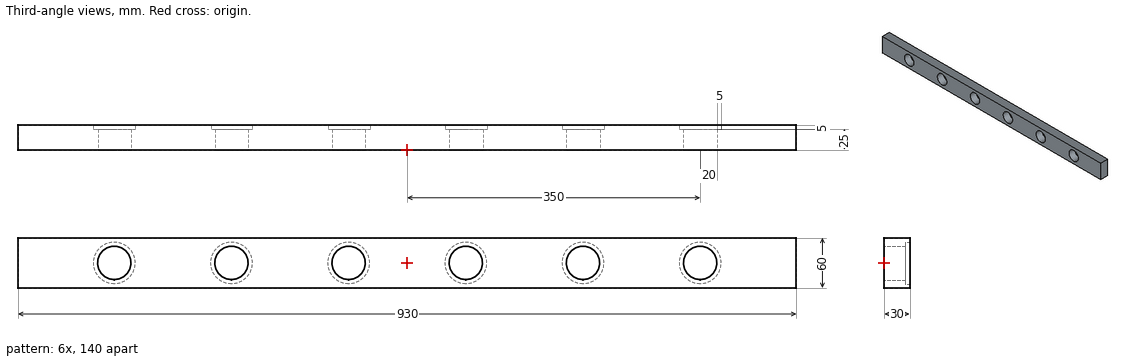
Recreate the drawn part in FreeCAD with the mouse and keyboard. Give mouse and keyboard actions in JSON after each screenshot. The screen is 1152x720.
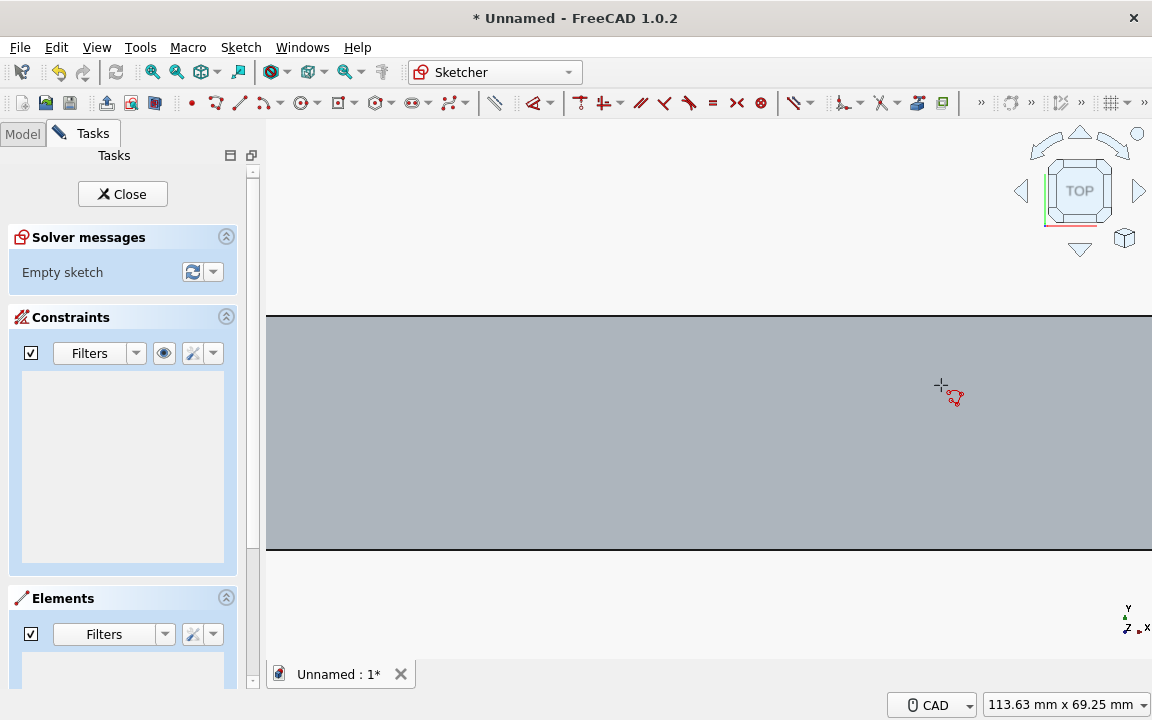
{"action": "left_click", "coordinate": [537, 550]}
{"action": "left_click", "coordinate": [693, 541]}
{"action": "left_click", "coordinate": [693, 355]}
{"action": "left_click", "coordinate": [732, 355]}
{"action": "left_click", "coordinate": [732, 316]}
{"action": "left_click", "coordinate": [537, 316]}
{"action": "left_click", "coordinate": [537, 551]}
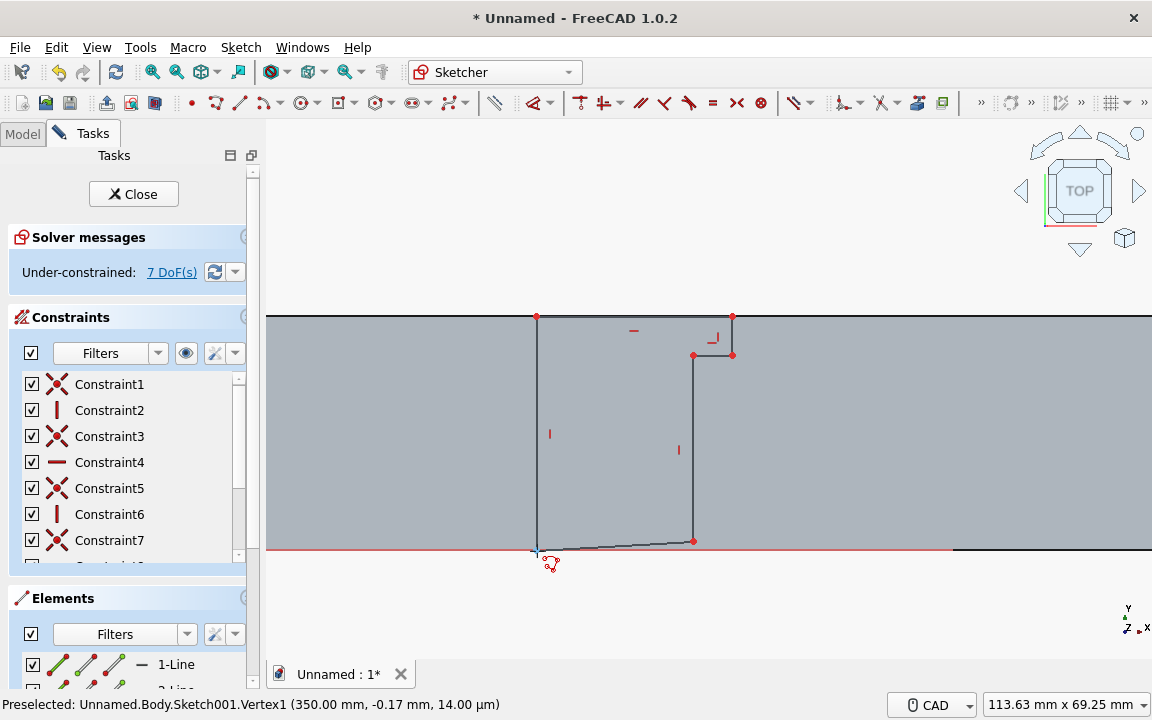
{"action": "key", "text": "g l"}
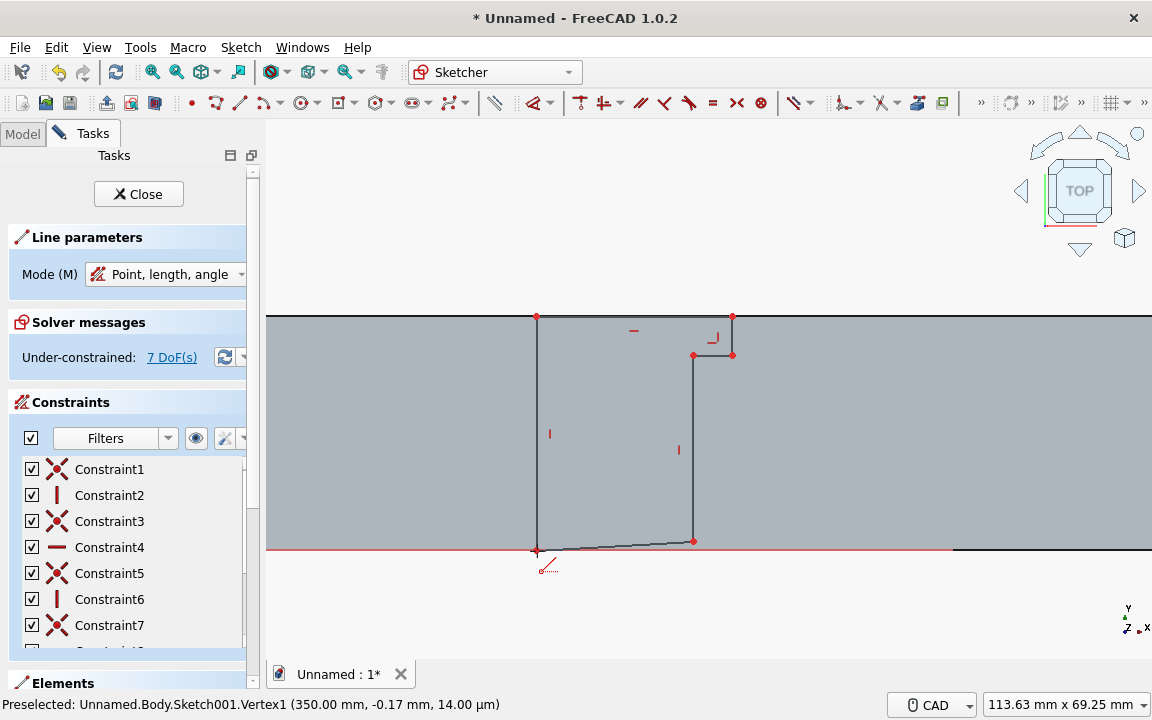
{"action": "left_click", "coordinate": [537, 292]}
{"action": "left_click", "coordinate": [537, 222]}
{"action": "key", "text": "Escape"}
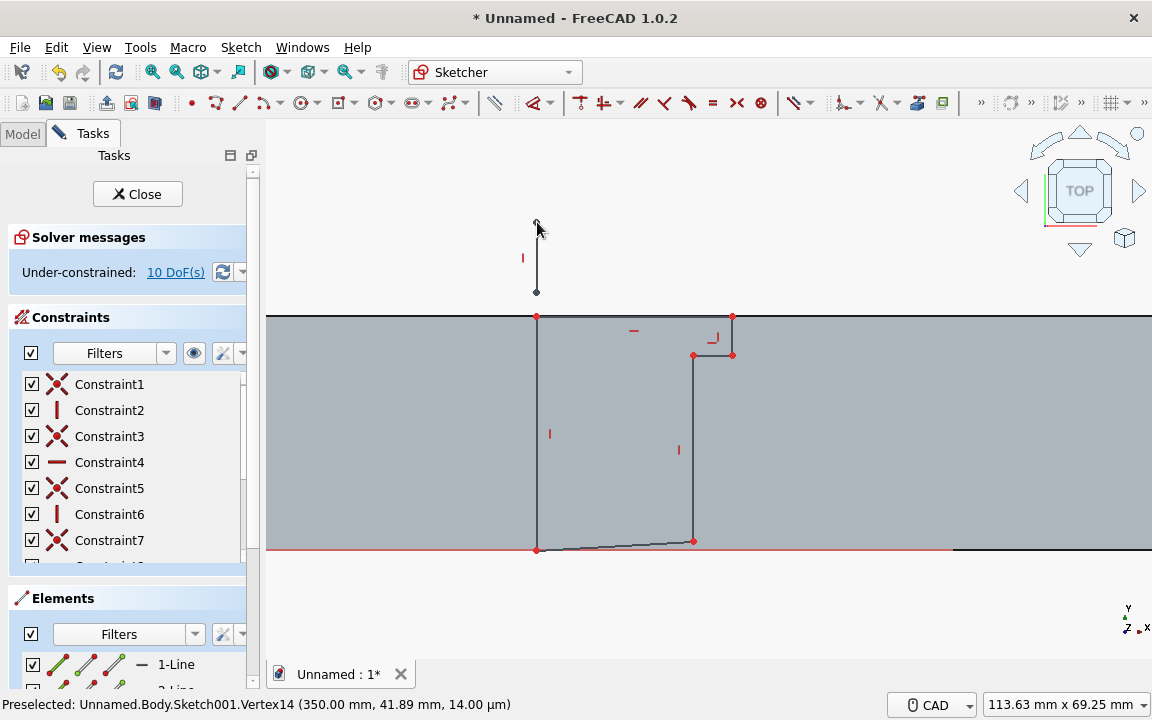
{"action": "left_click", "coordinate": [537, 272]}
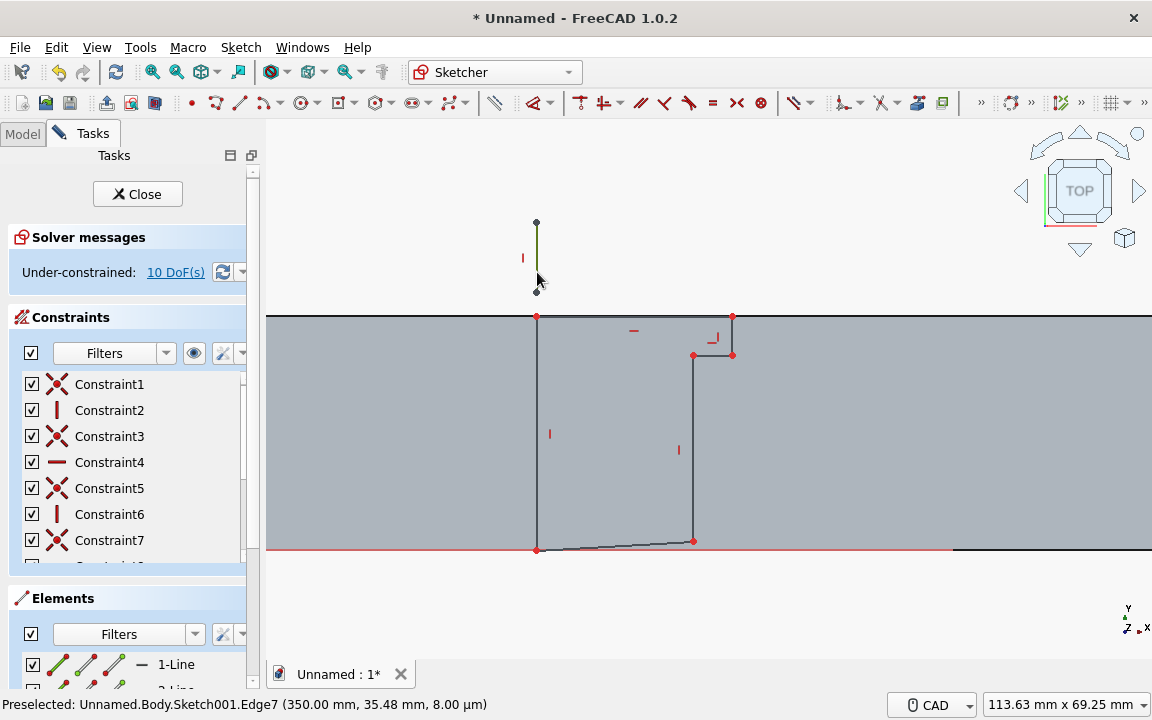
{"action": "left_click", "coordinate": [496, 104]}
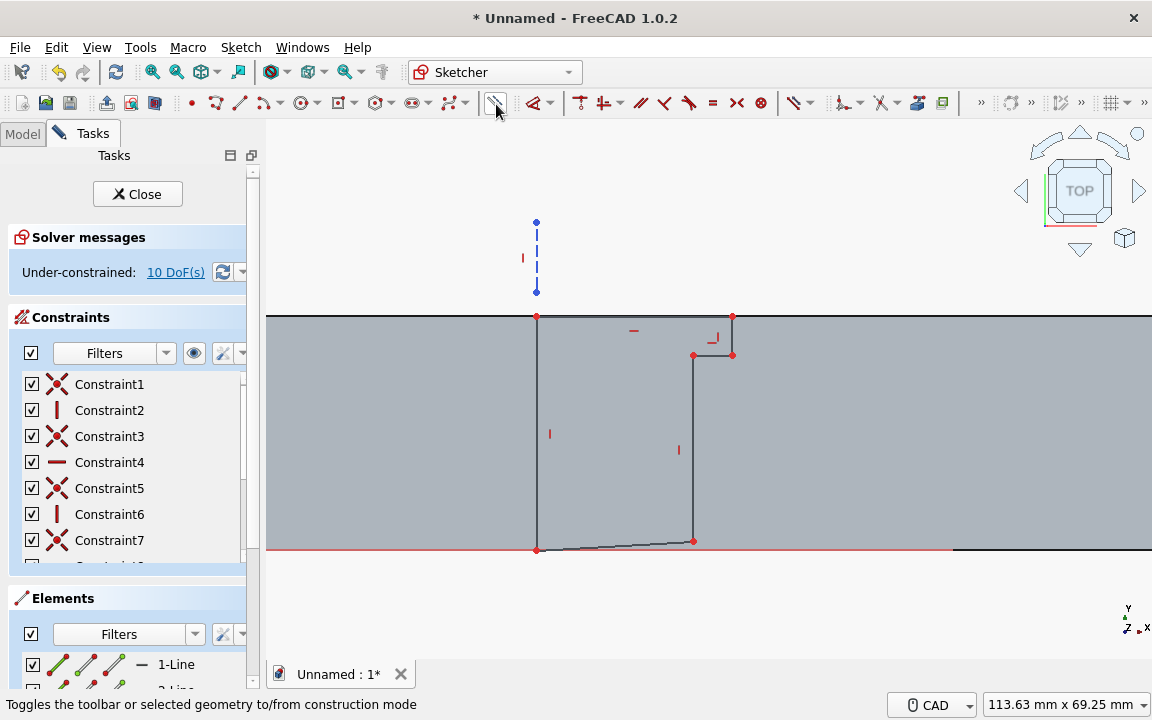
{"action": "left_click", "coordinate": [584, 548]}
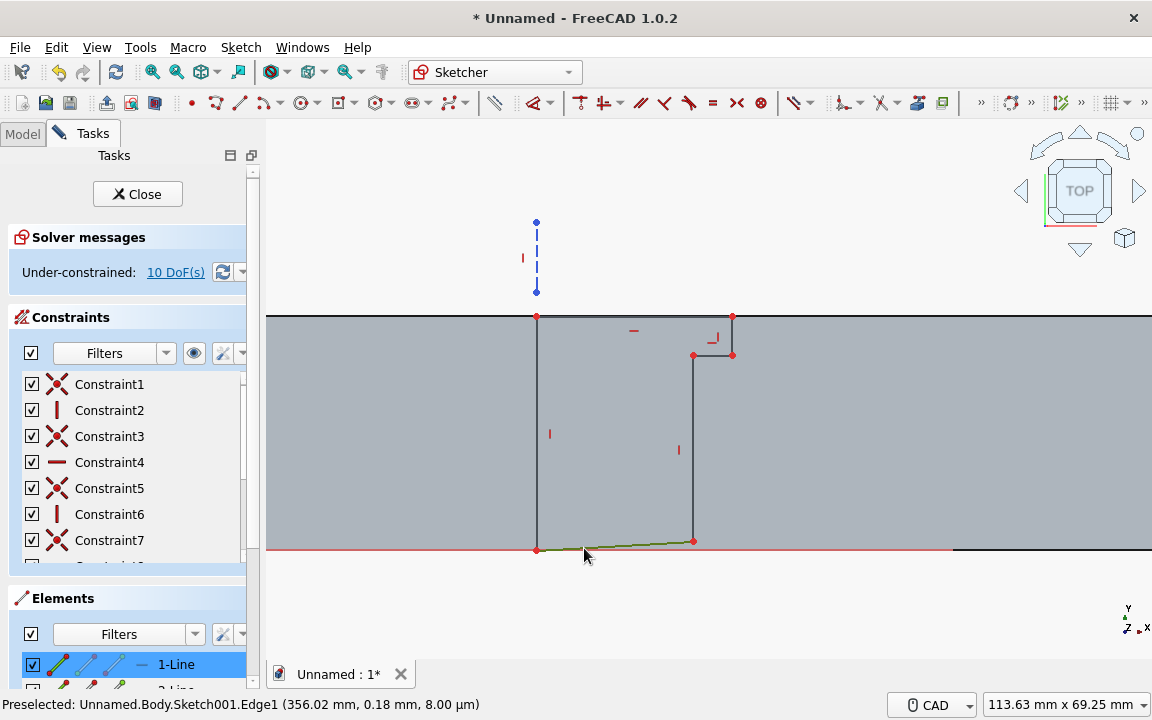
{"action": "key", "text": "h"}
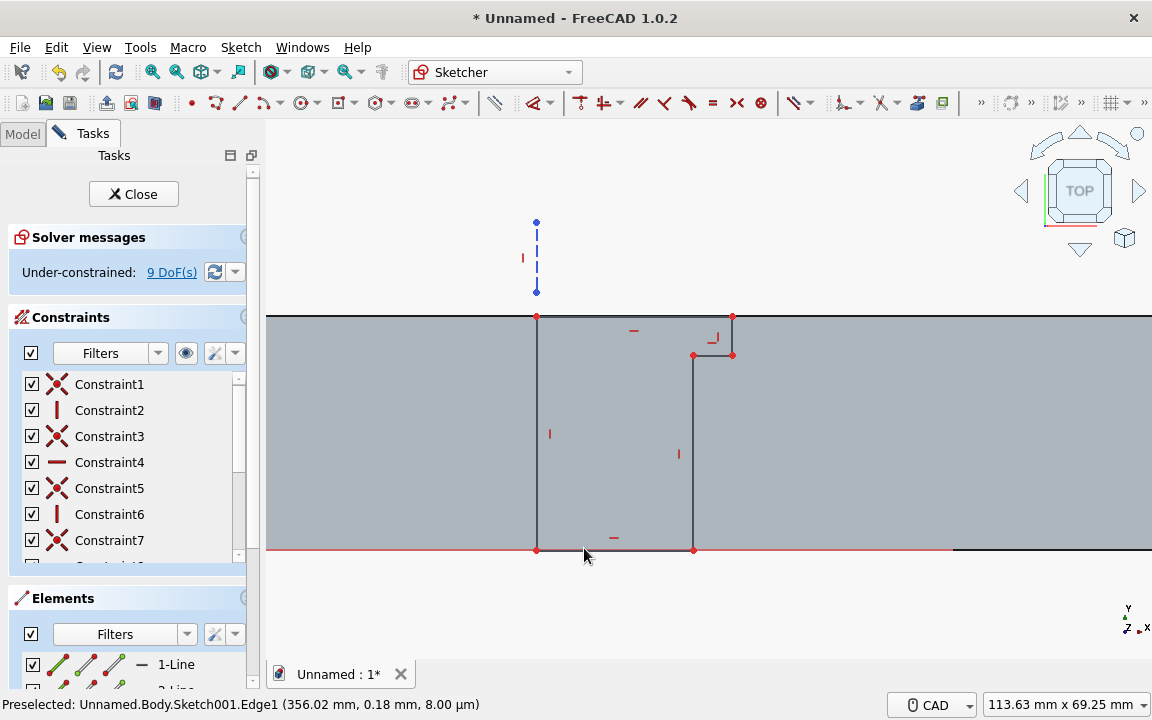
{"action": "left_click", "coordinate": [537, 551]}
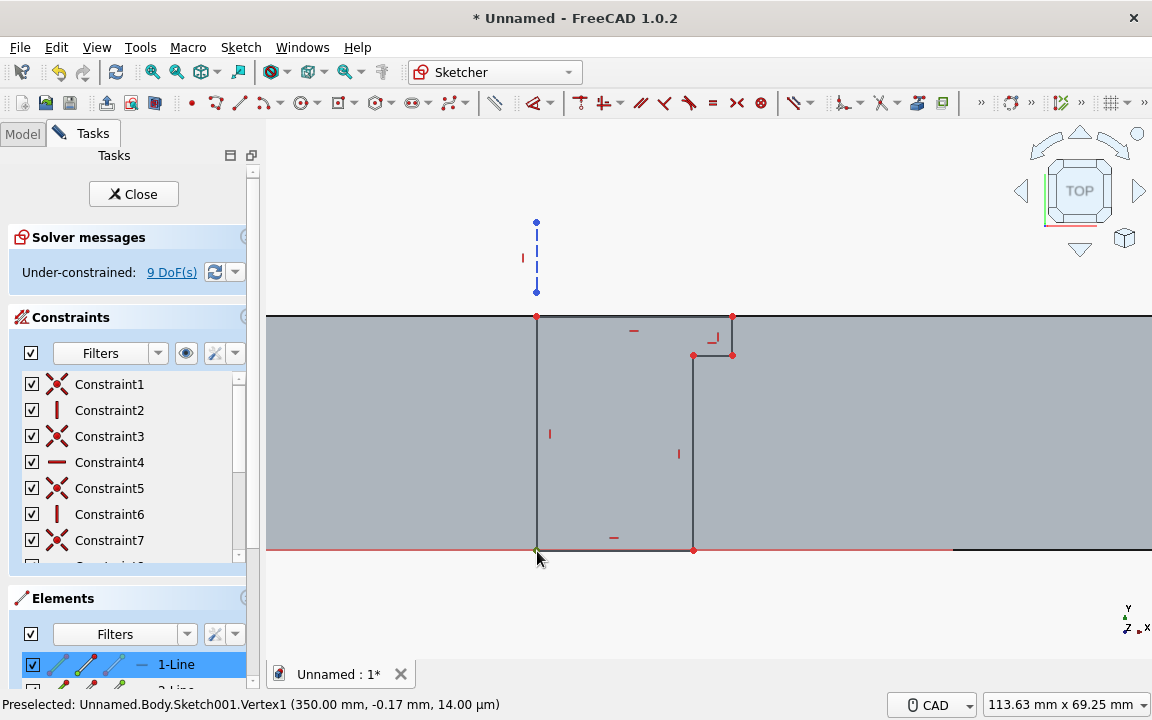
{"action": "left_click", "coordinate": [344, 550]}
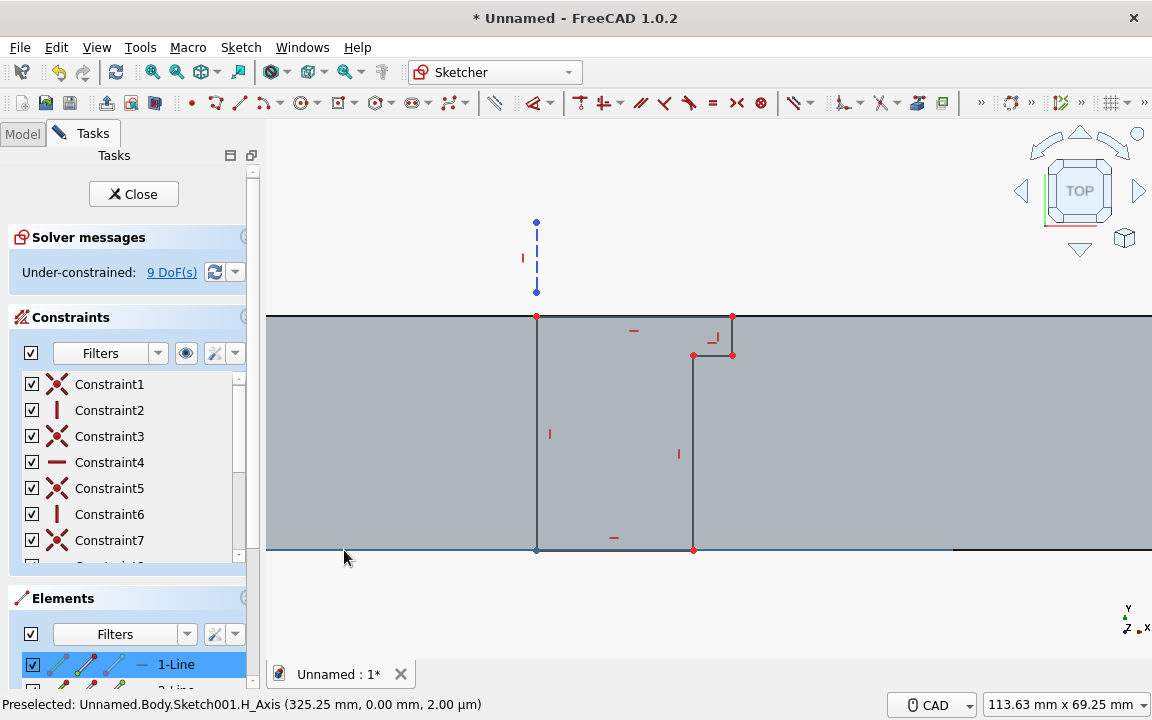
{"action": "left_click", "coordinate": [580, 104]}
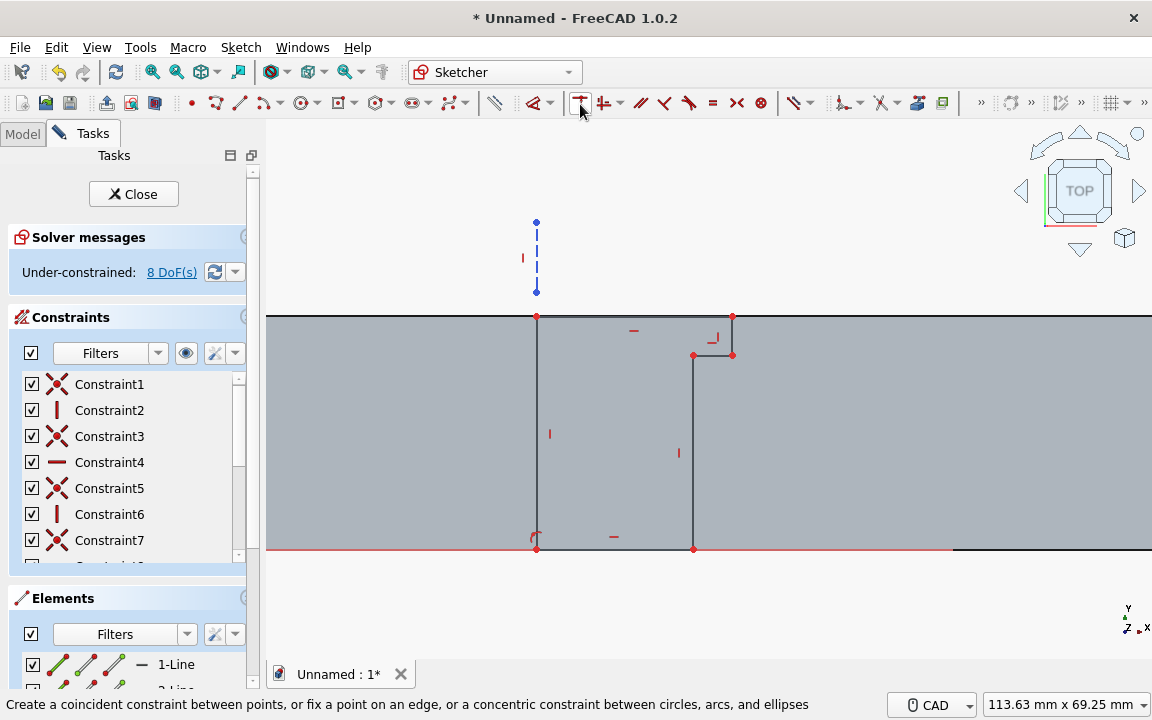
{"action": "left_click", "coordinate": [534, 104]}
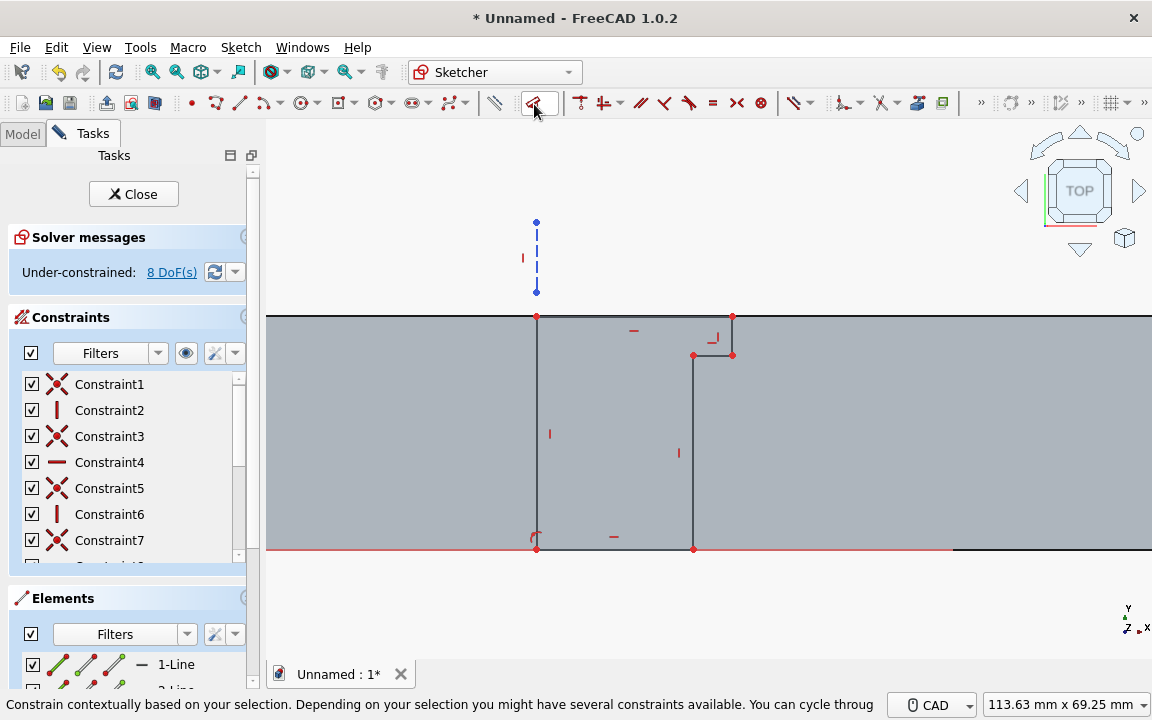
{"action": "left_click", "coordinate": [705, 356]}
{"action": "left_click", "coordinate": [712, 390]}